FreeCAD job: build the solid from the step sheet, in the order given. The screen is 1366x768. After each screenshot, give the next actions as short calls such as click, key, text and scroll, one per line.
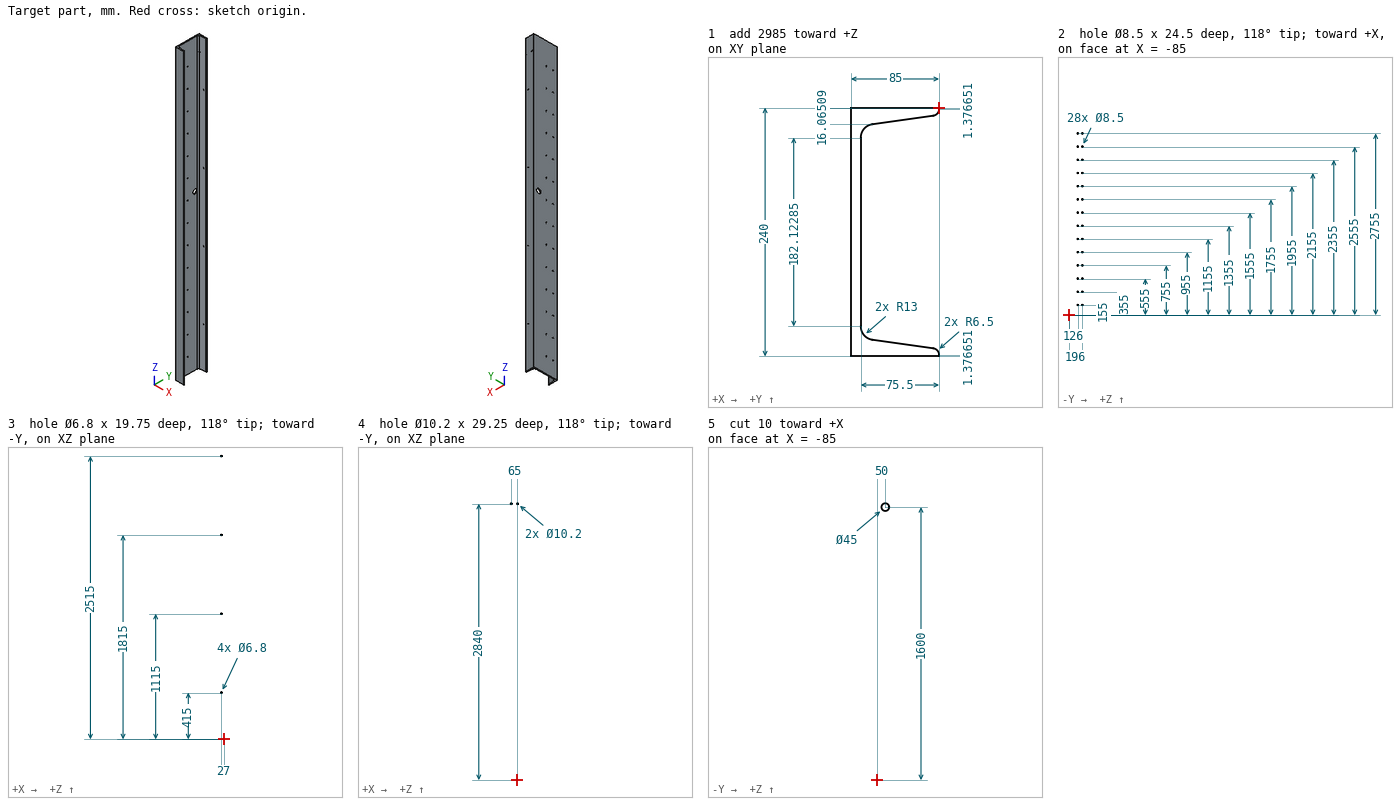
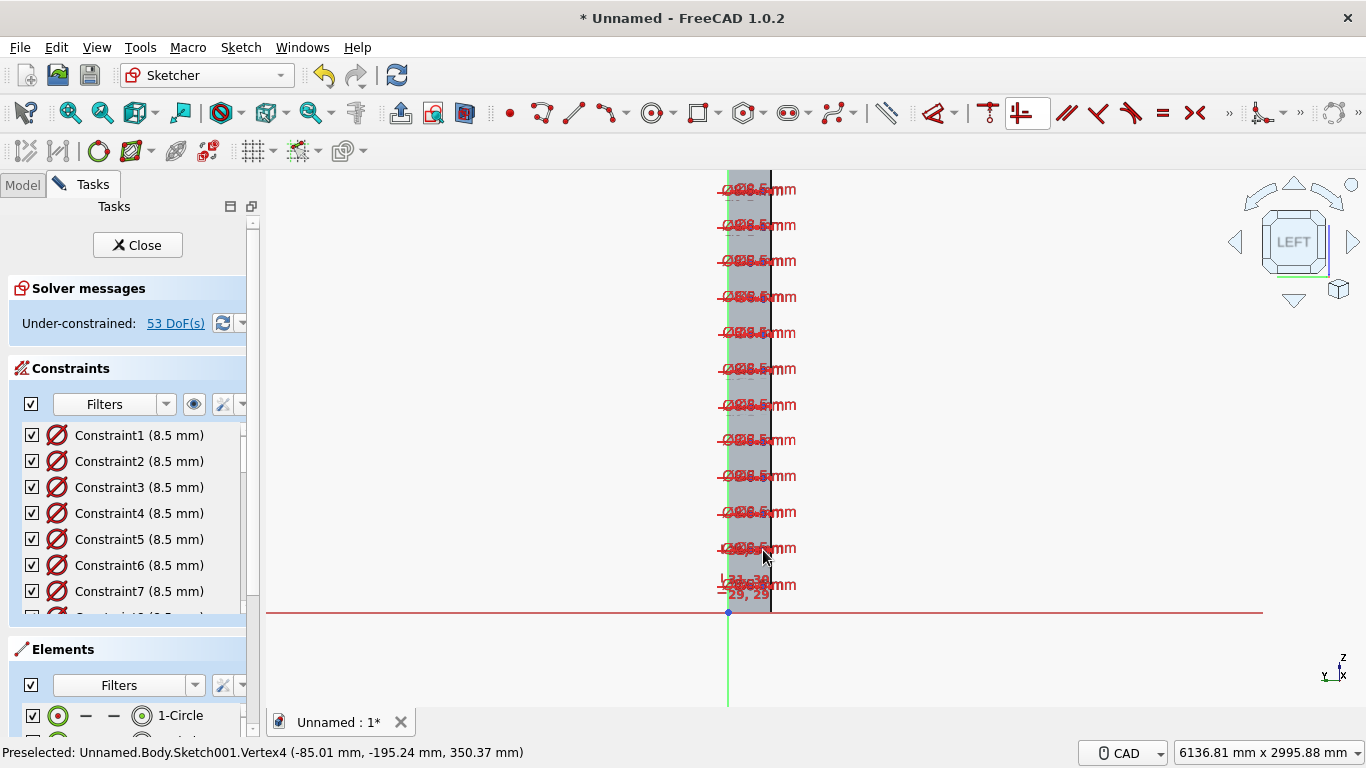
scroll(750, 551, up, 4)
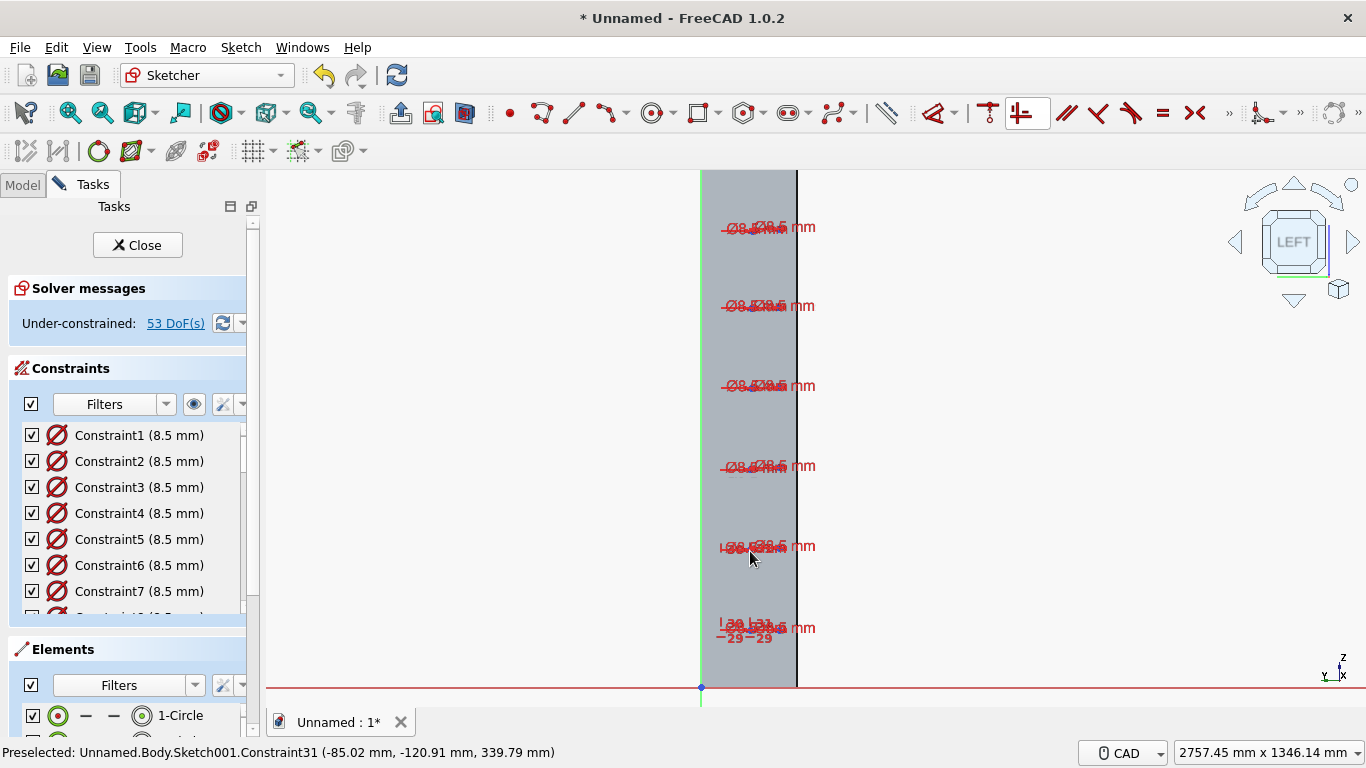
scroll(751, 550, up, 4)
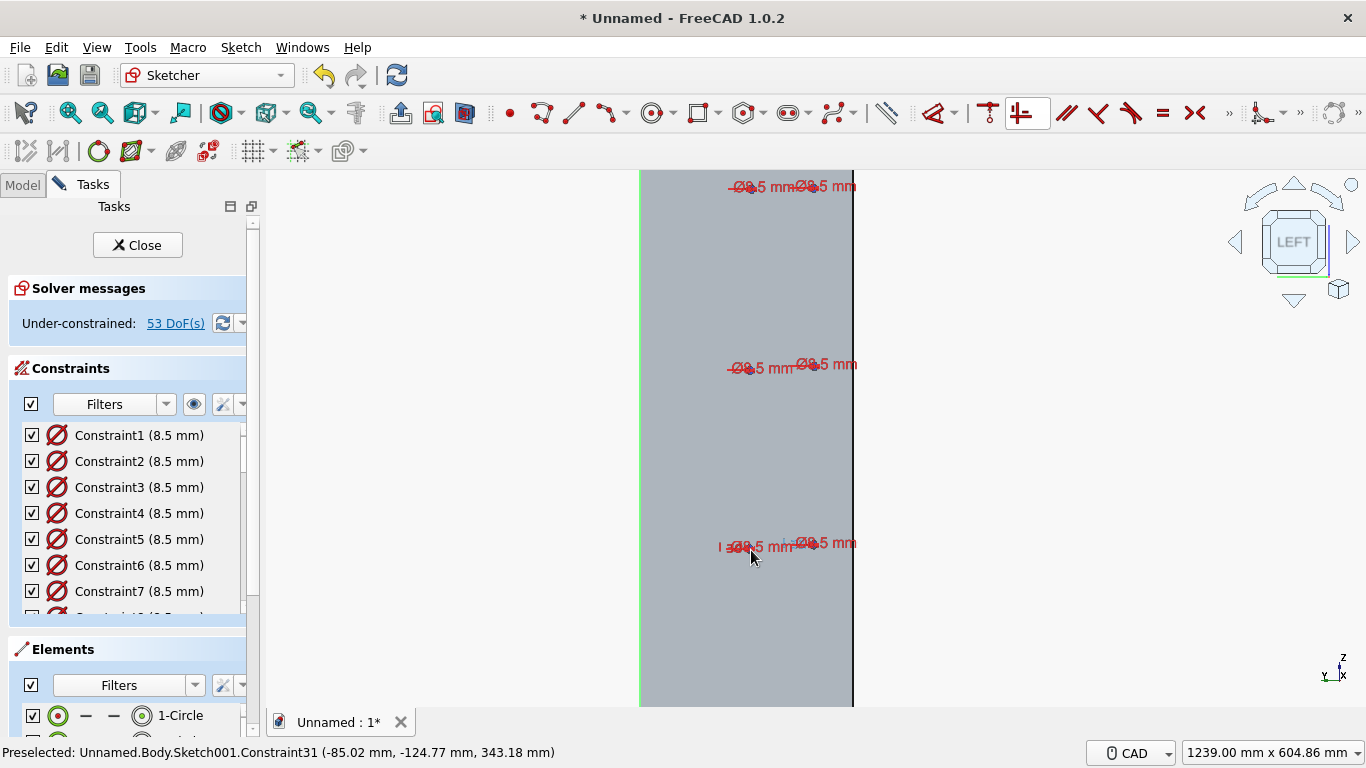
click(750, 549)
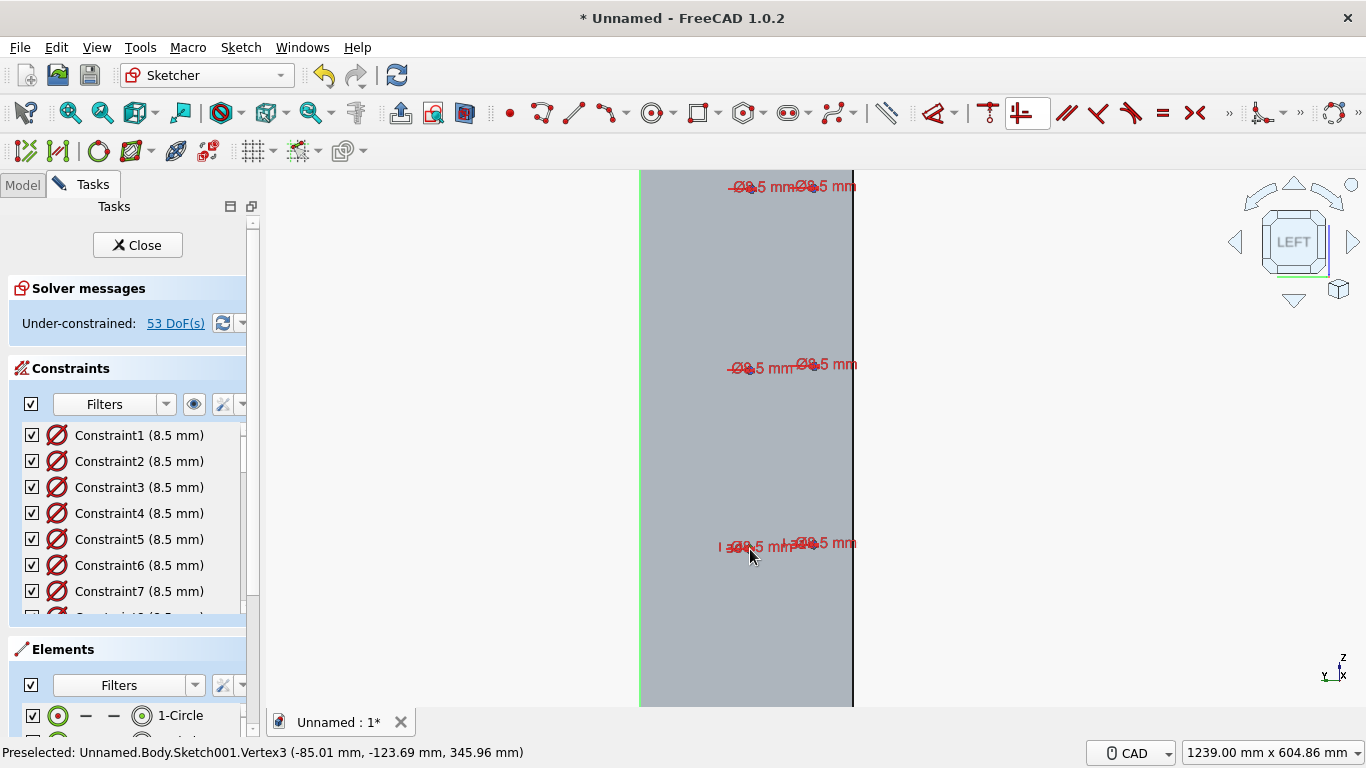
scroll(750, 565, down, 10)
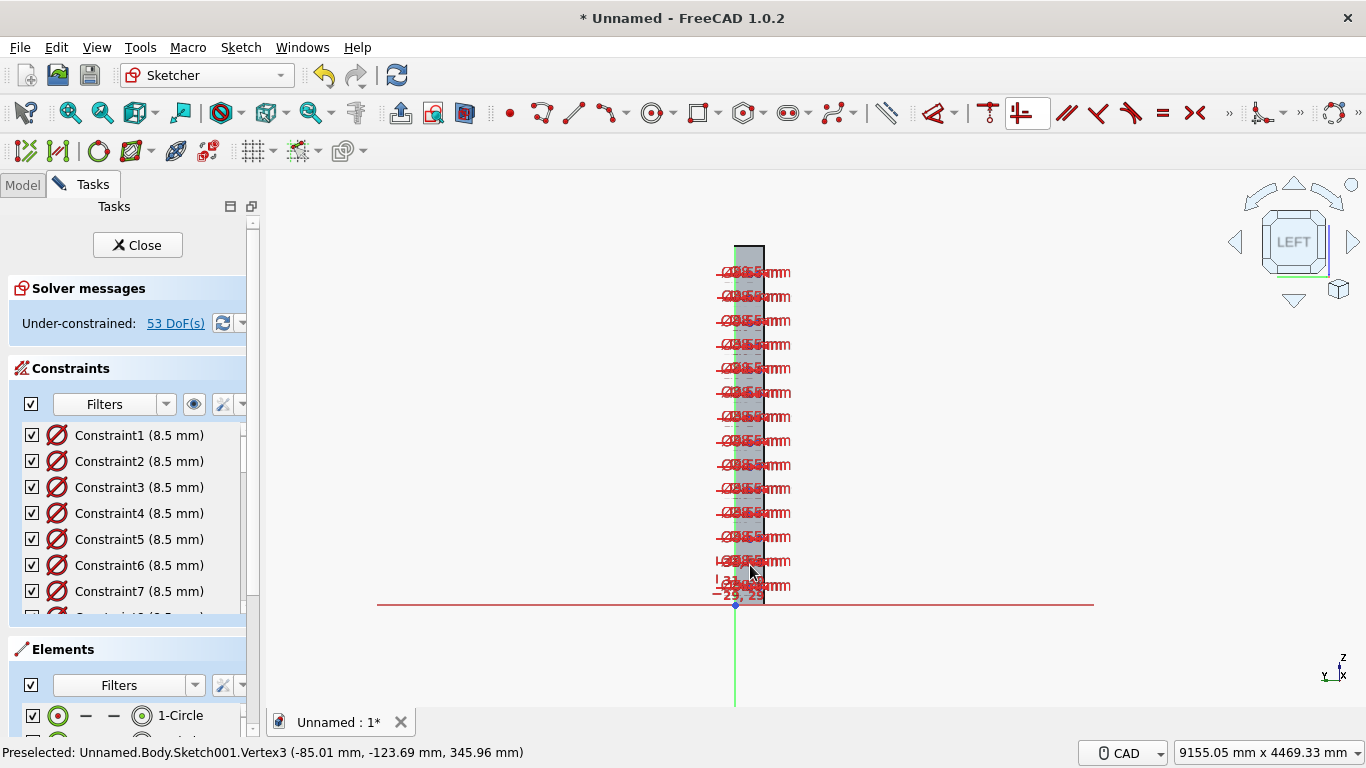
scroll(759, 563, up, 2)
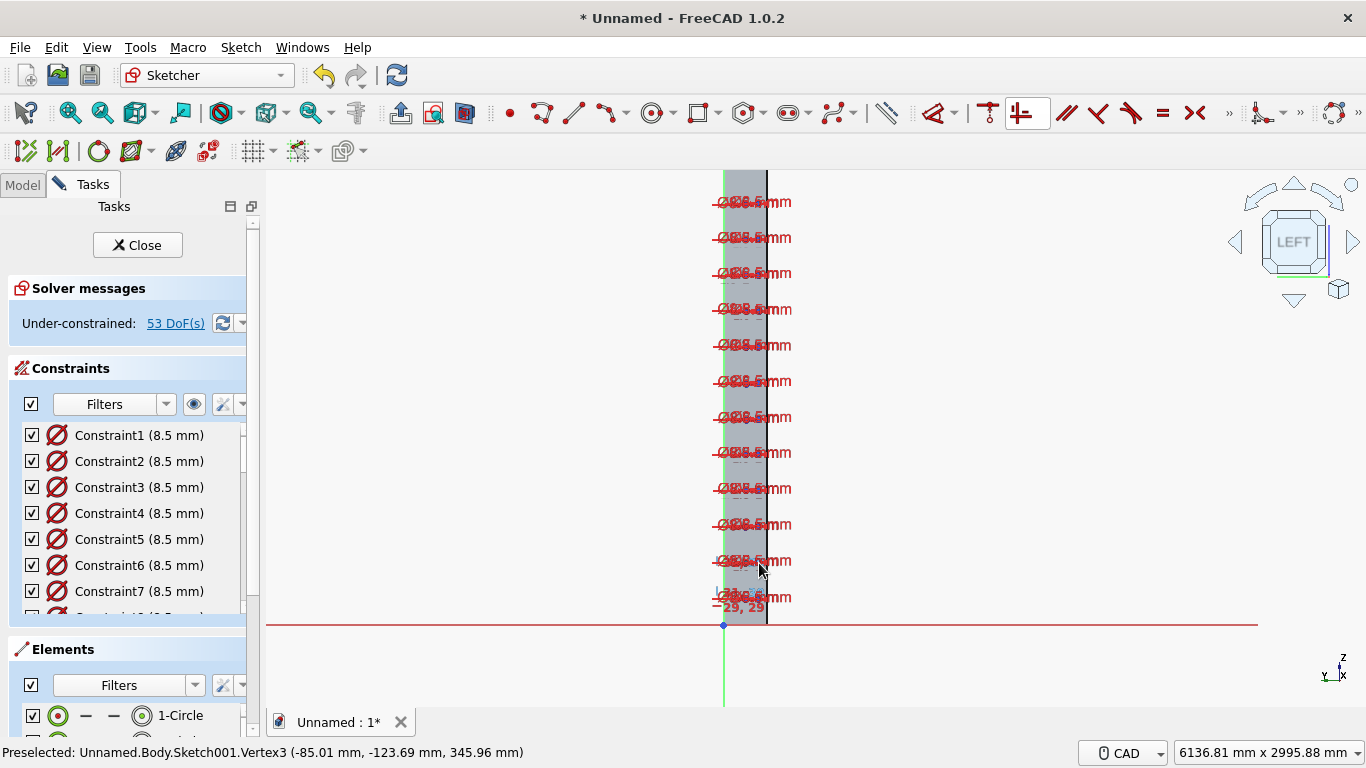
scroll(759, 563, up, 4)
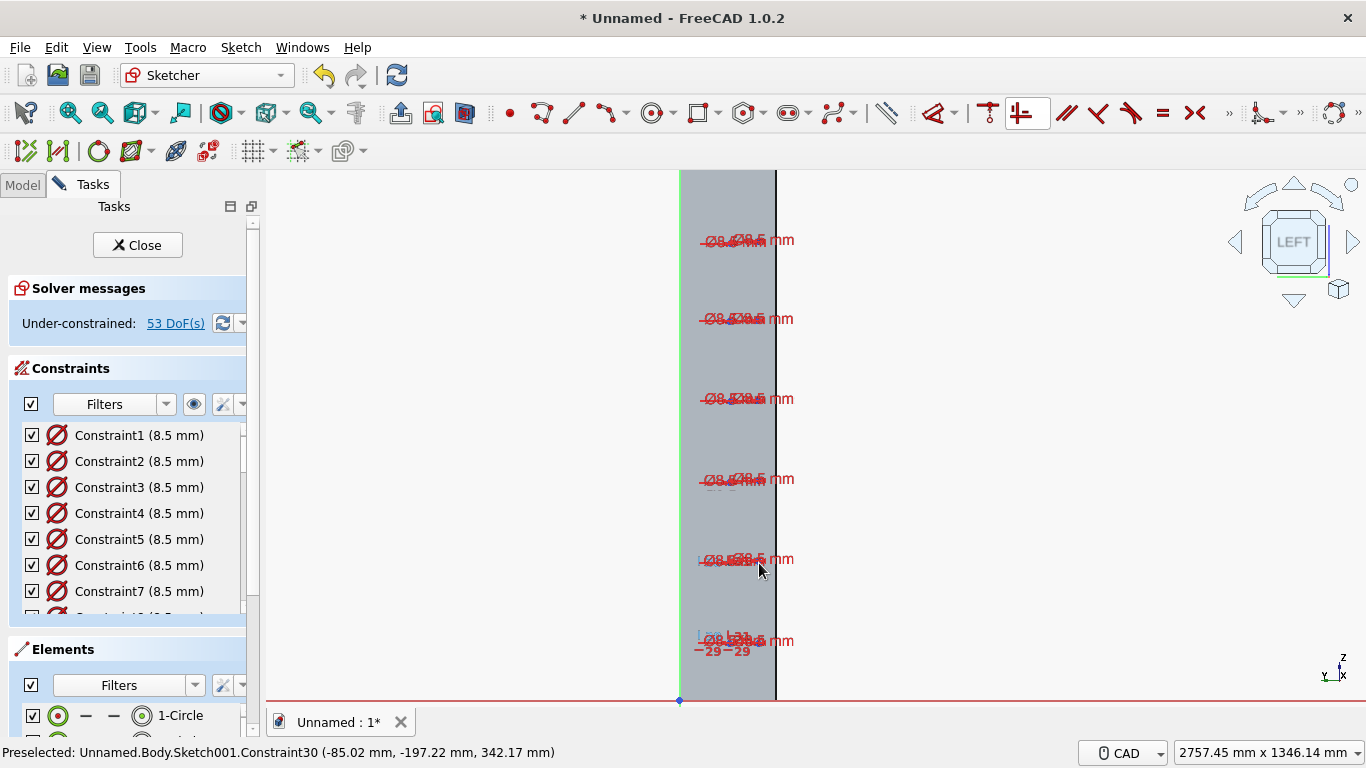
click(758, 561)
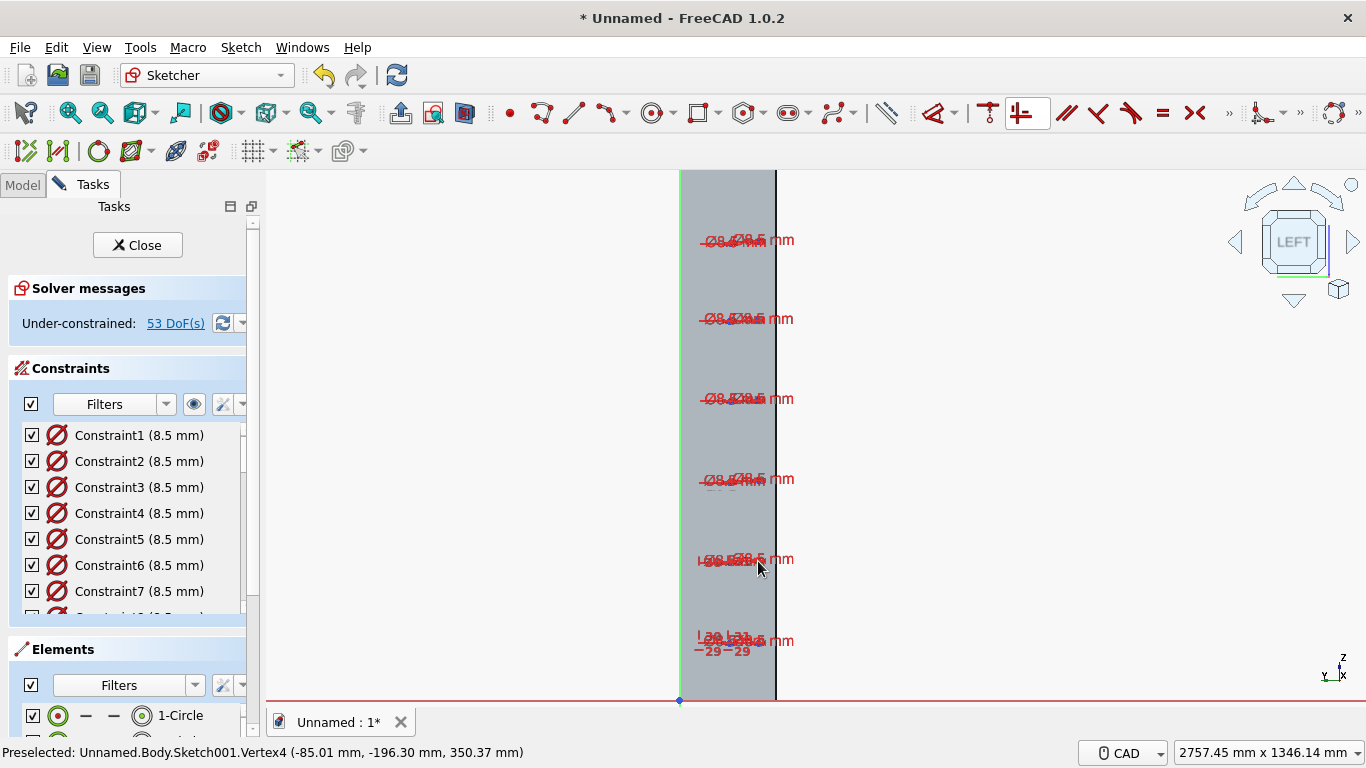
click(1044, 114)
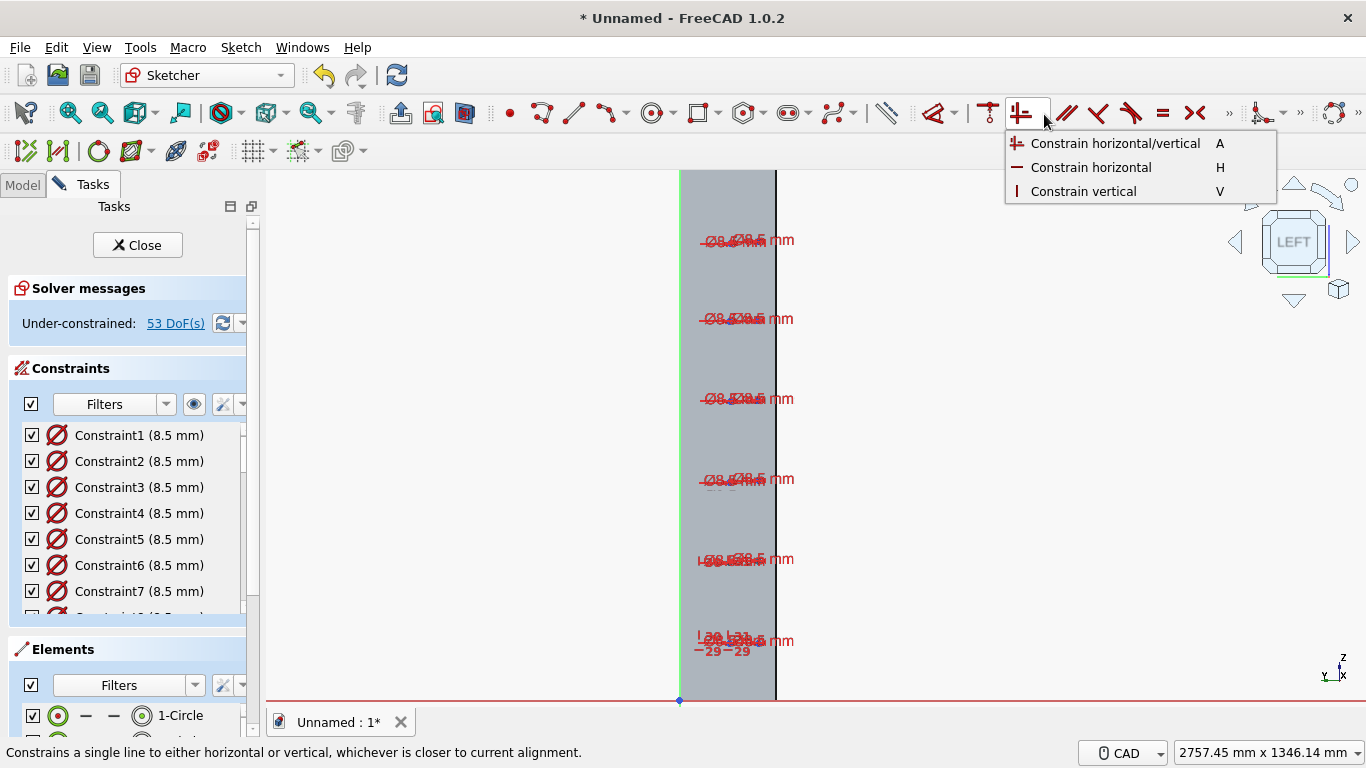
click(1141, 167)